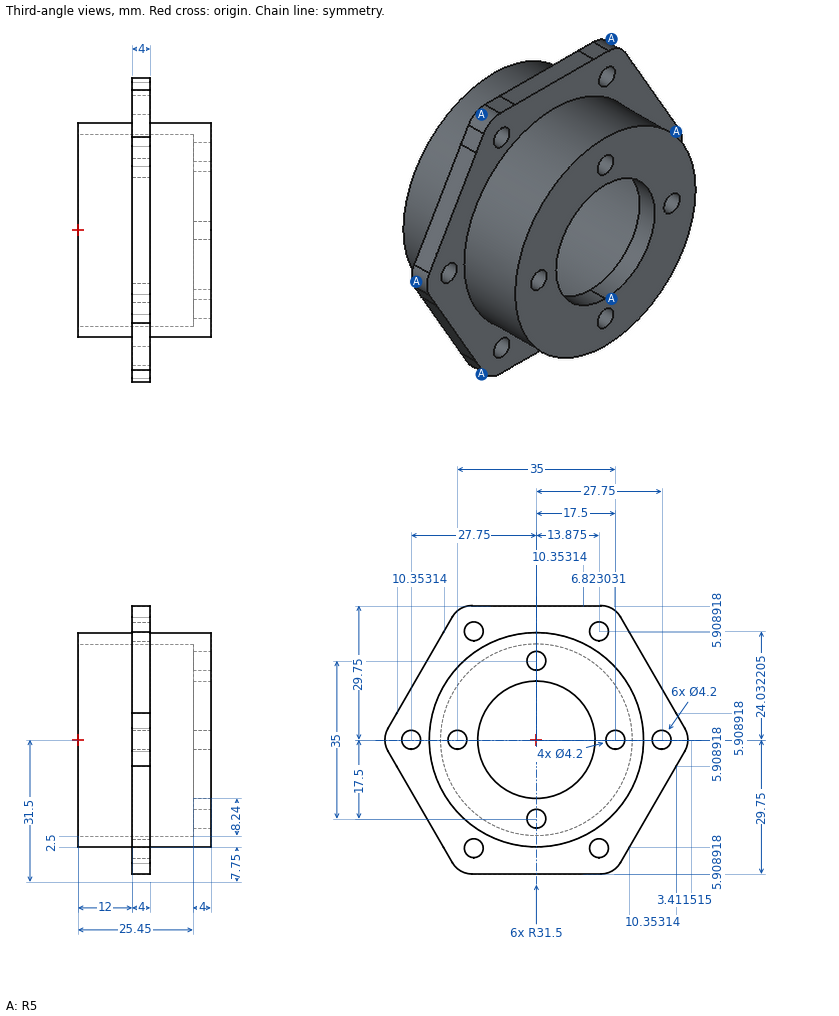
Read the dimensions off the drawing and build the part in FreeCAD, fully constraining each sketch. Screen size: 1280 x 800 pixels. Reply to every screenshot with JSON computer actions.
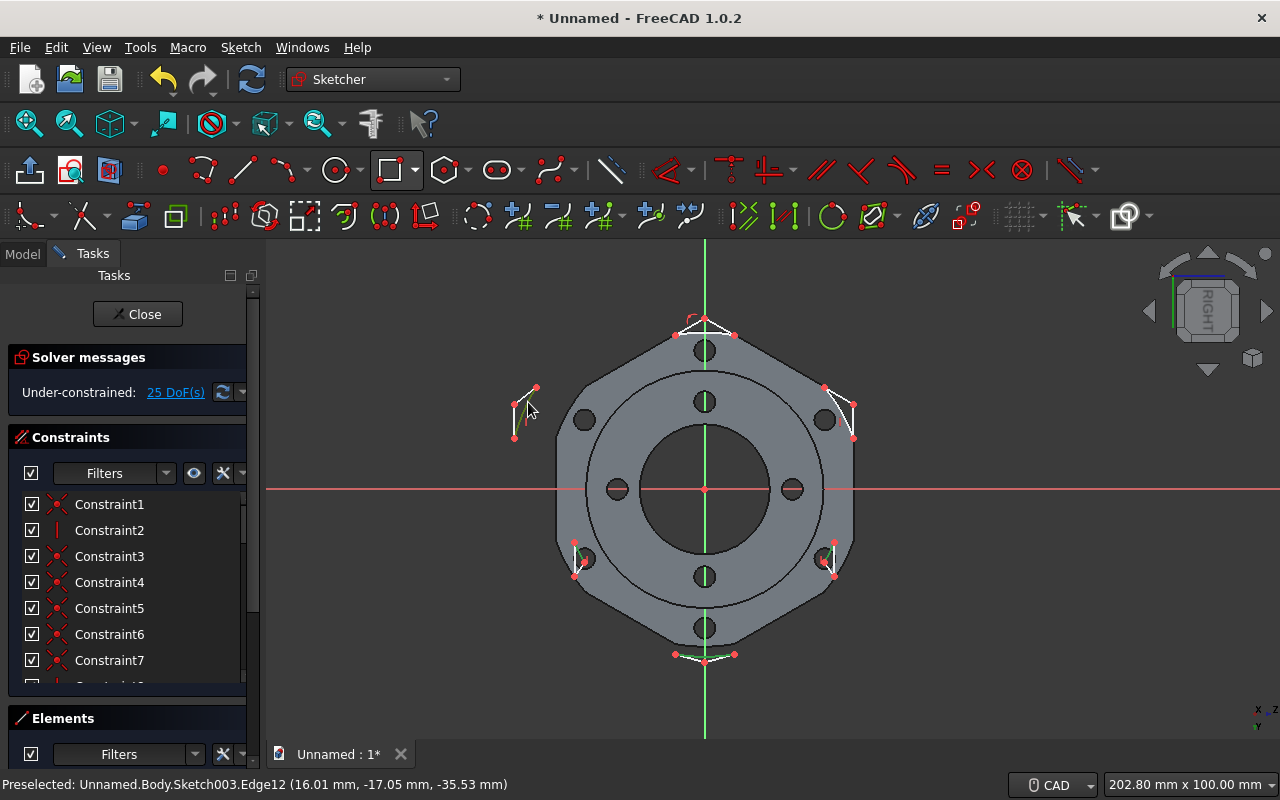
{"action": "scroll", "coordinate": [717, 333], "scroll_direction": "up", "scroll_amount": 4}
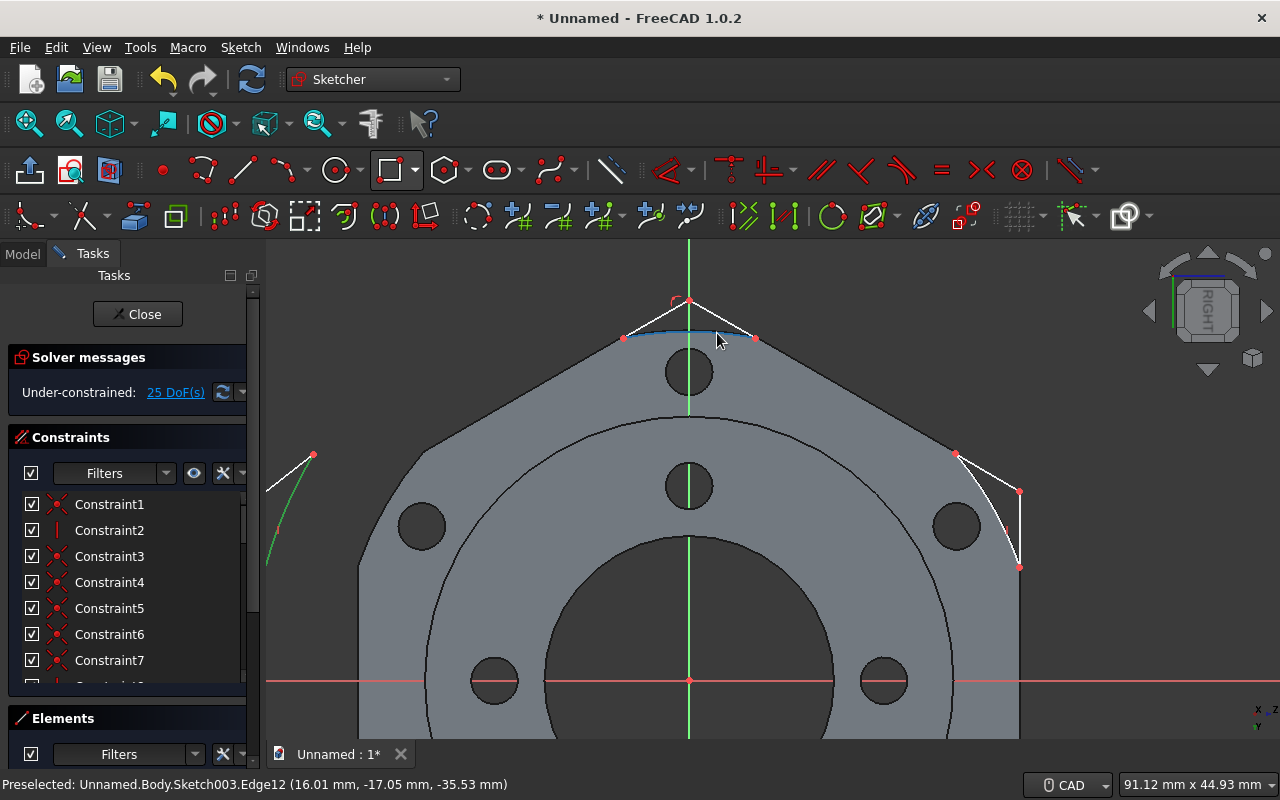
{"action": "left_click", "coordinate": [716, 333]}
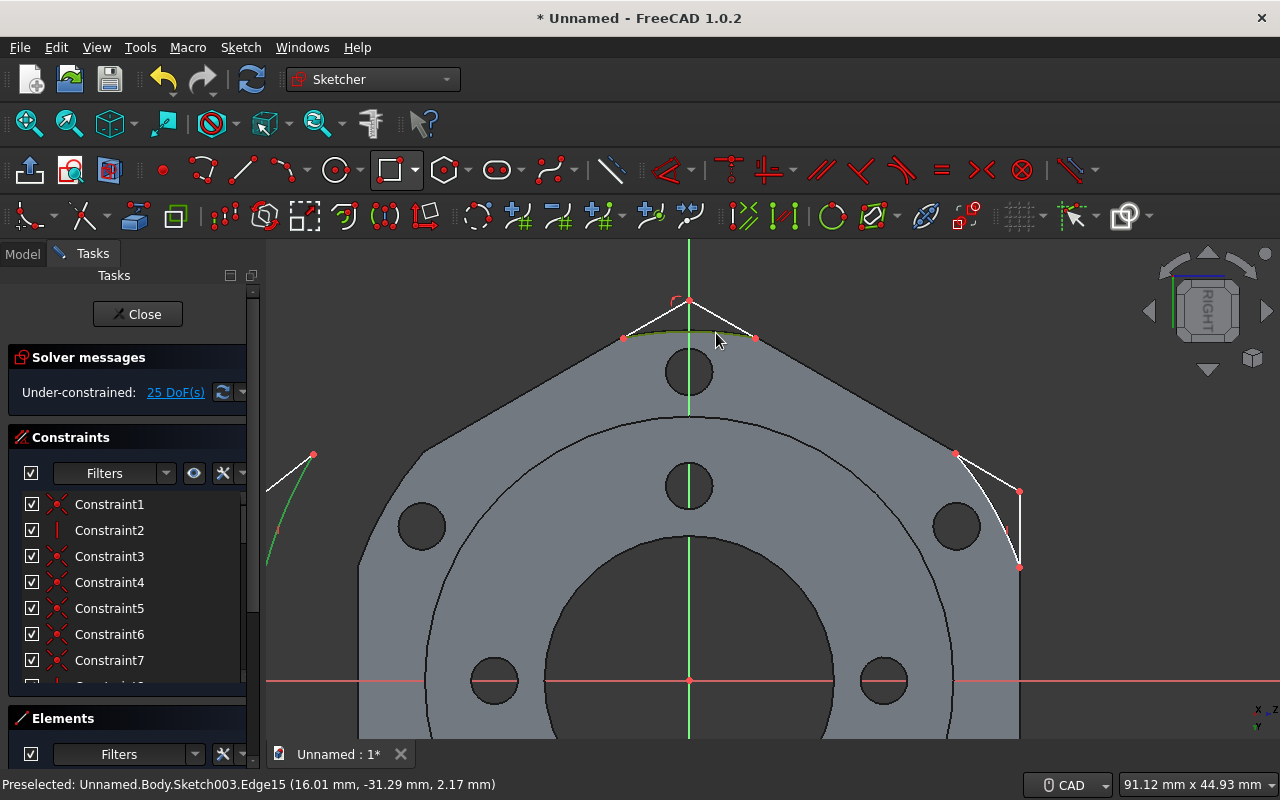
{"action": "left_click", "coordinate": [979, 485]}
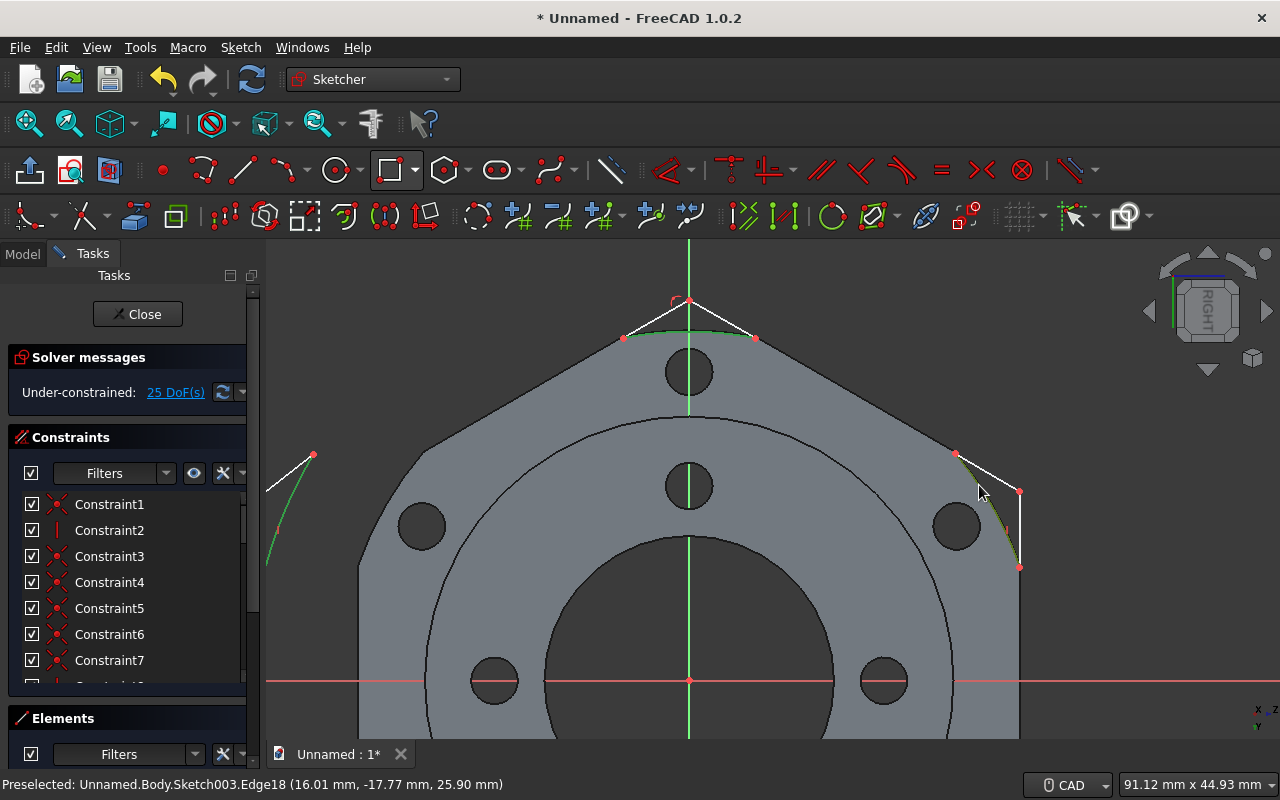
{"action": "key", "text": "e"}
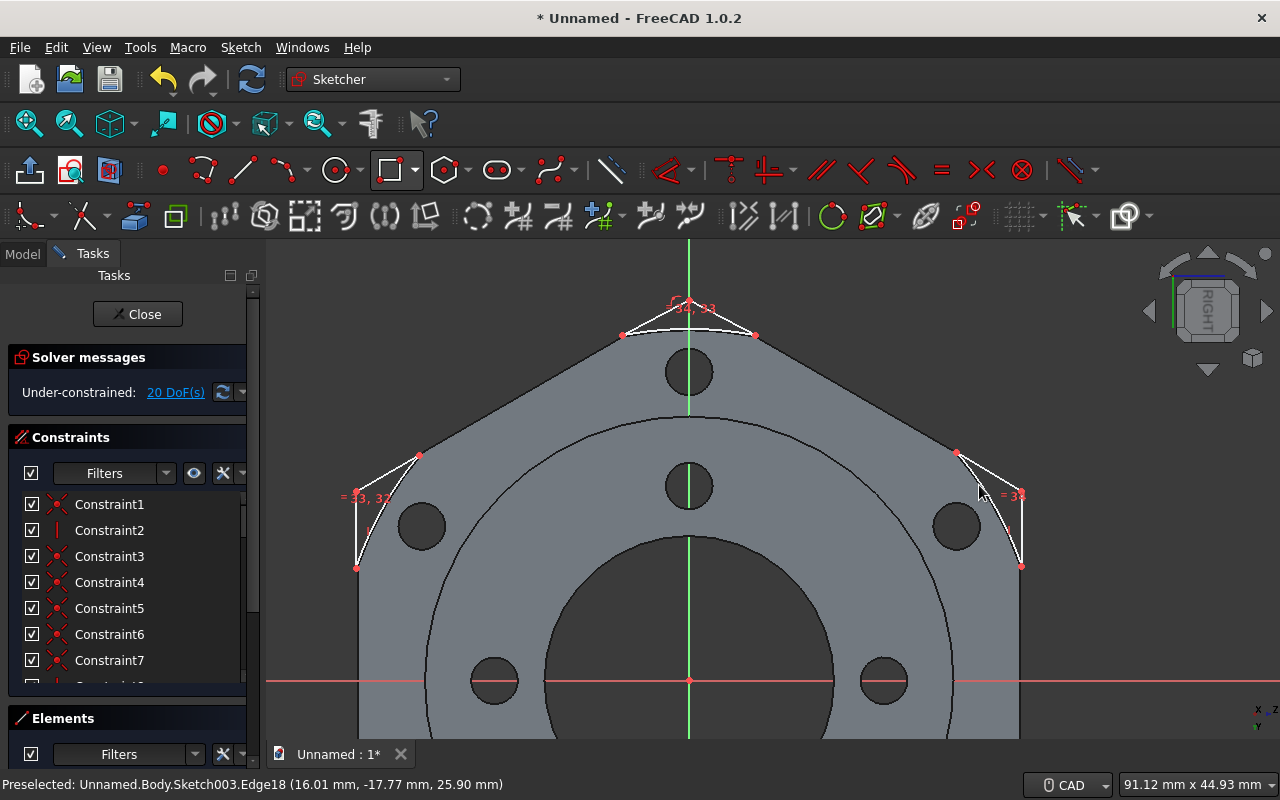
{"action": "scroll", "coordinate": [717, 333], "scroll_direction": "down", "scroll_amount": 4}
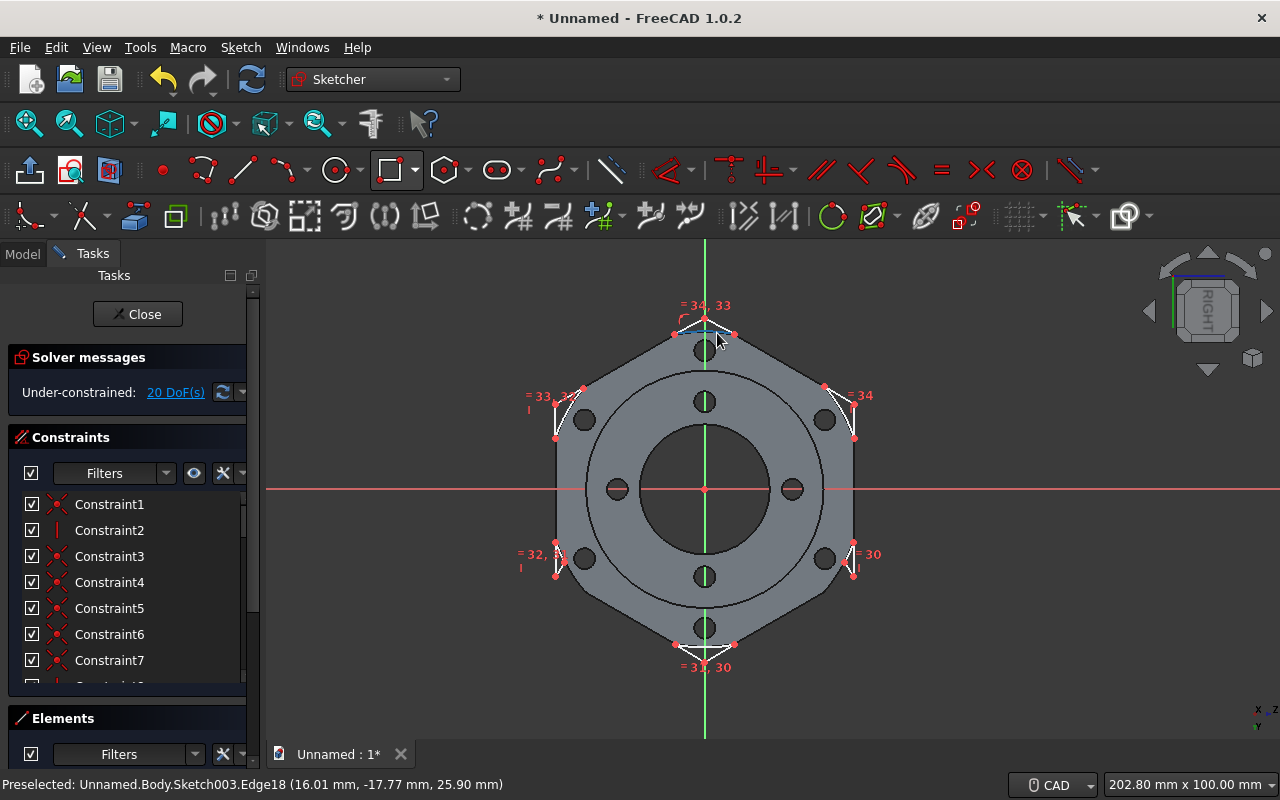
{"action": "left_click", "coordinate": [854, 576]}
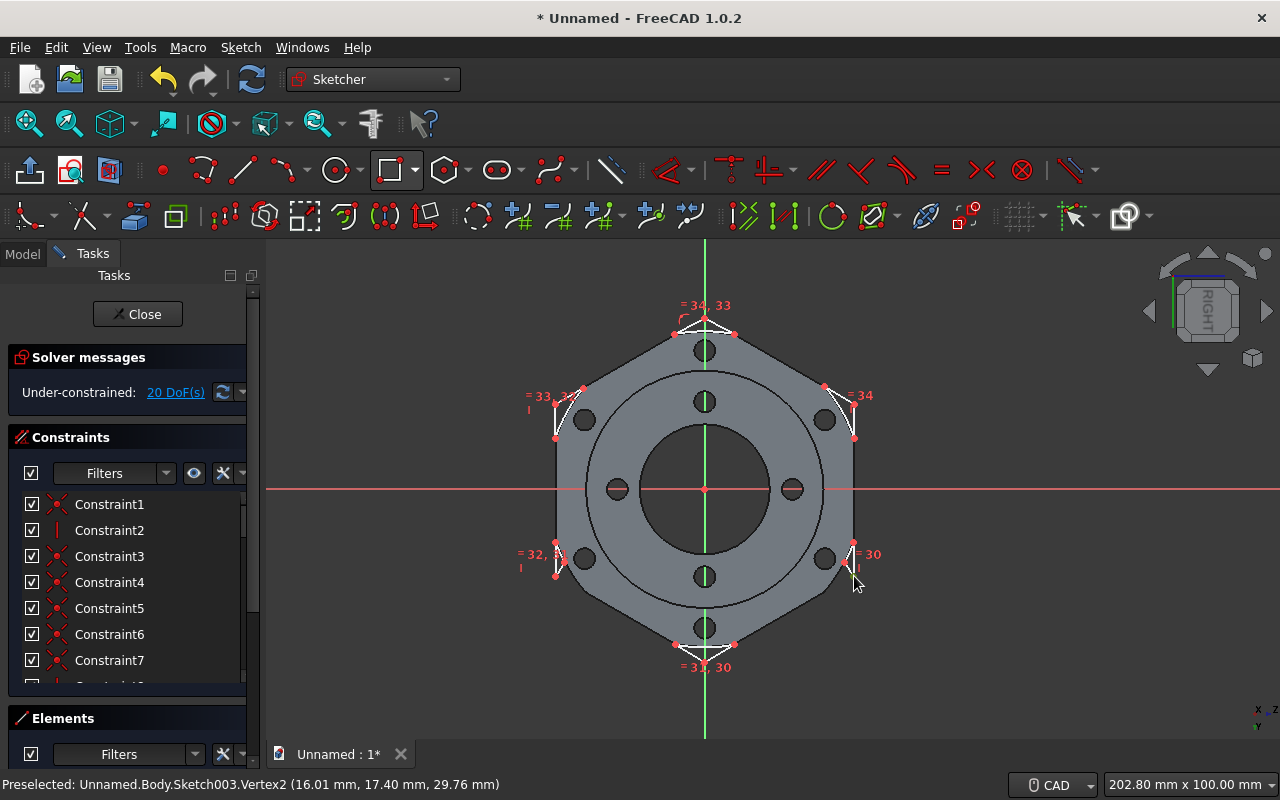
{"action": "left_click", "coordinate": [556, 577]}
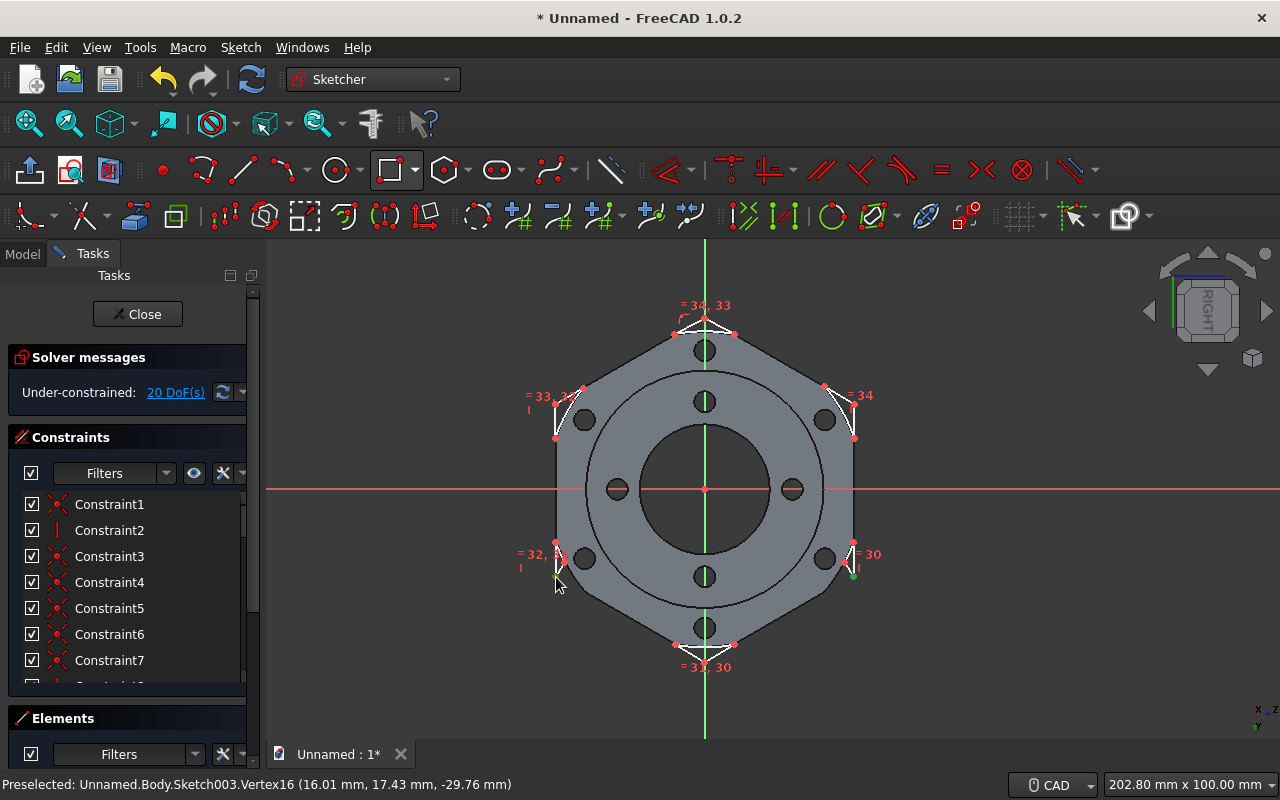
{"action": "left_click", "coordinate": [705, 616]}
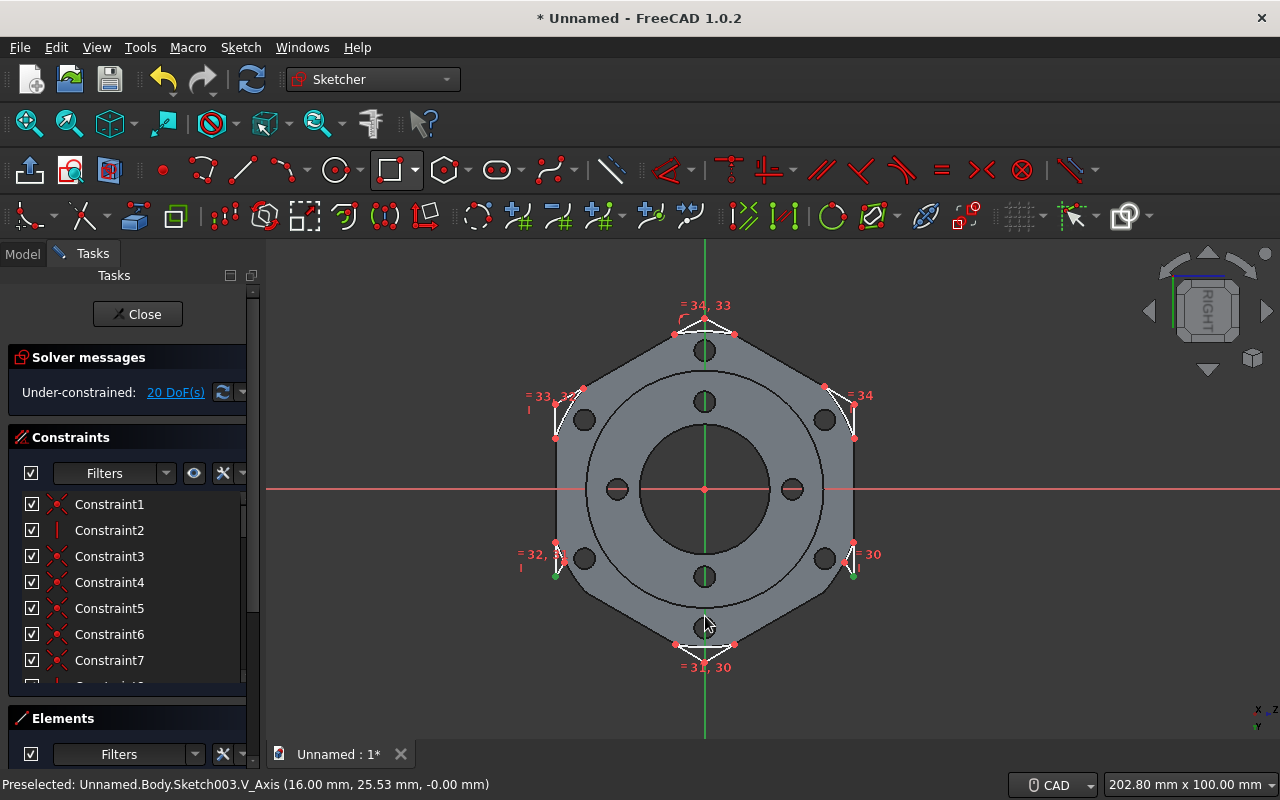
{"action": "key", "text": "s"}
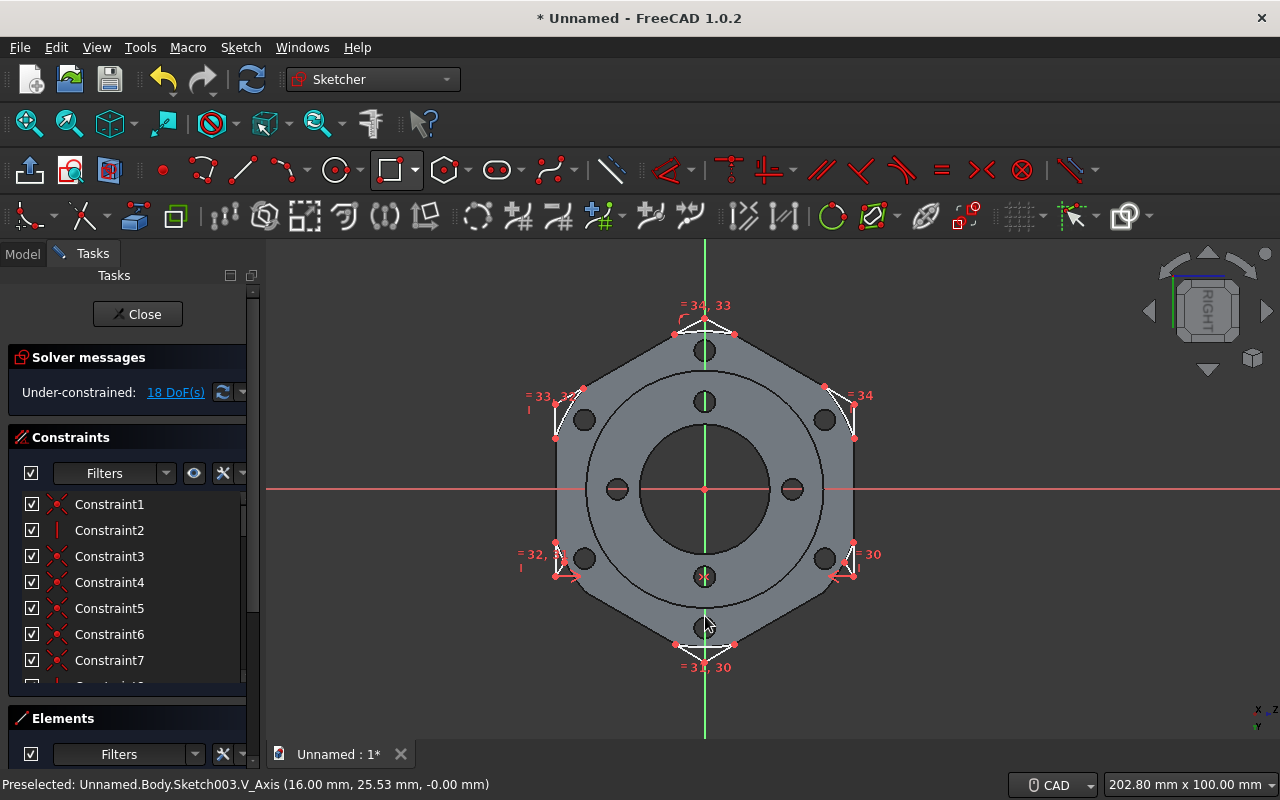
{"action": "left_click", "coordinate": [556, 576]}